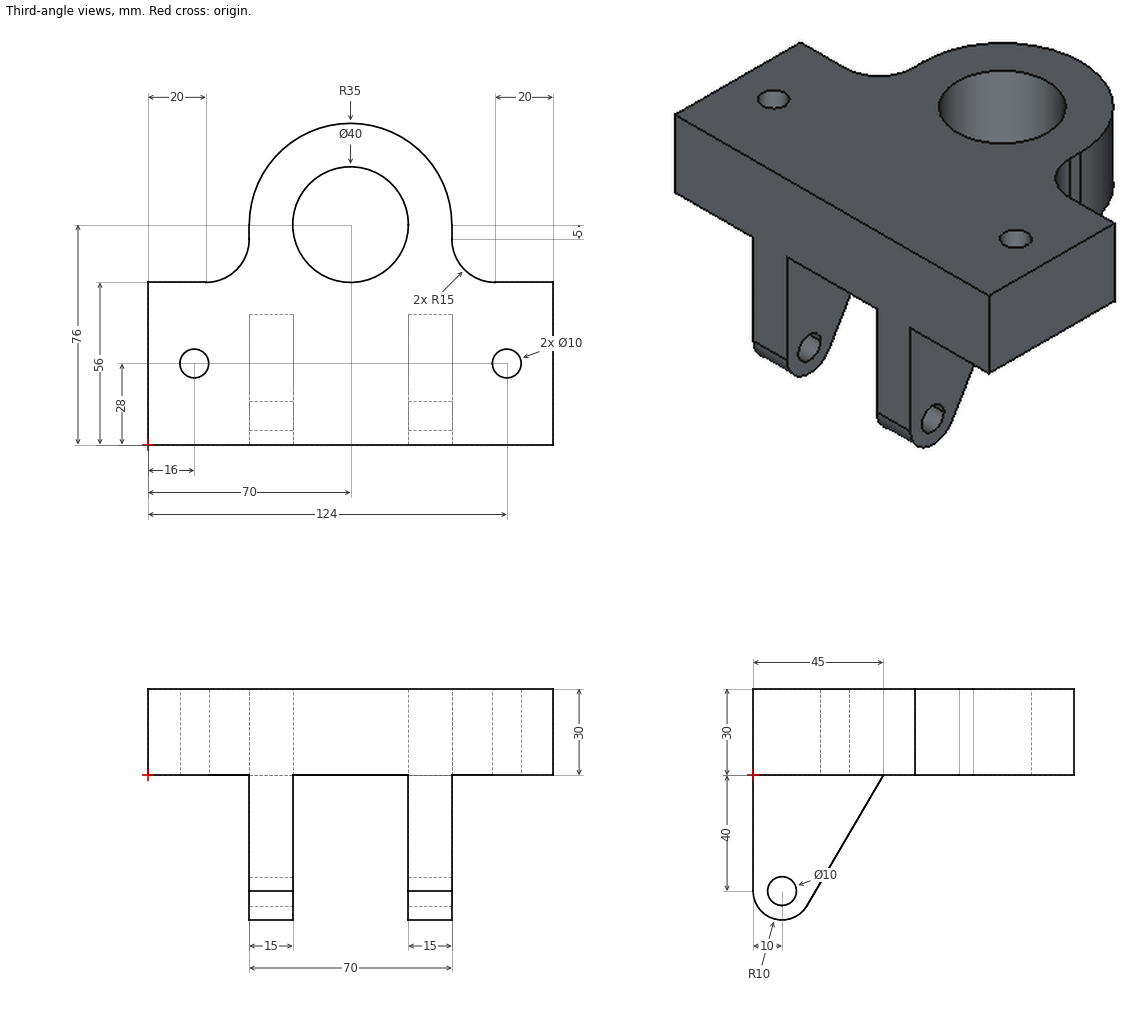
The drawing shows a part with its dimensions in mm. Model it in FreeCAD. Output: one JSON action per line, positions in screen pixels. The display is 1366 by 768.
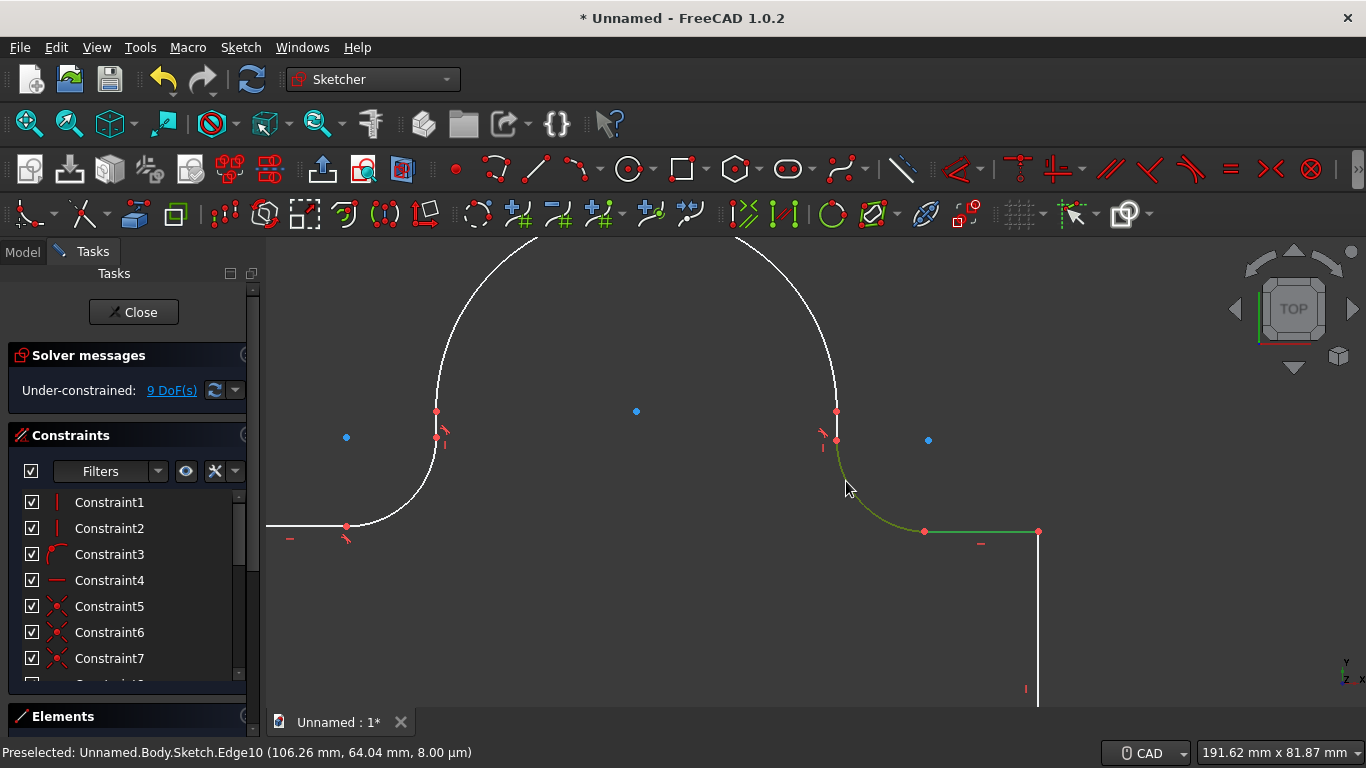
{"action": "key", "text": "t"}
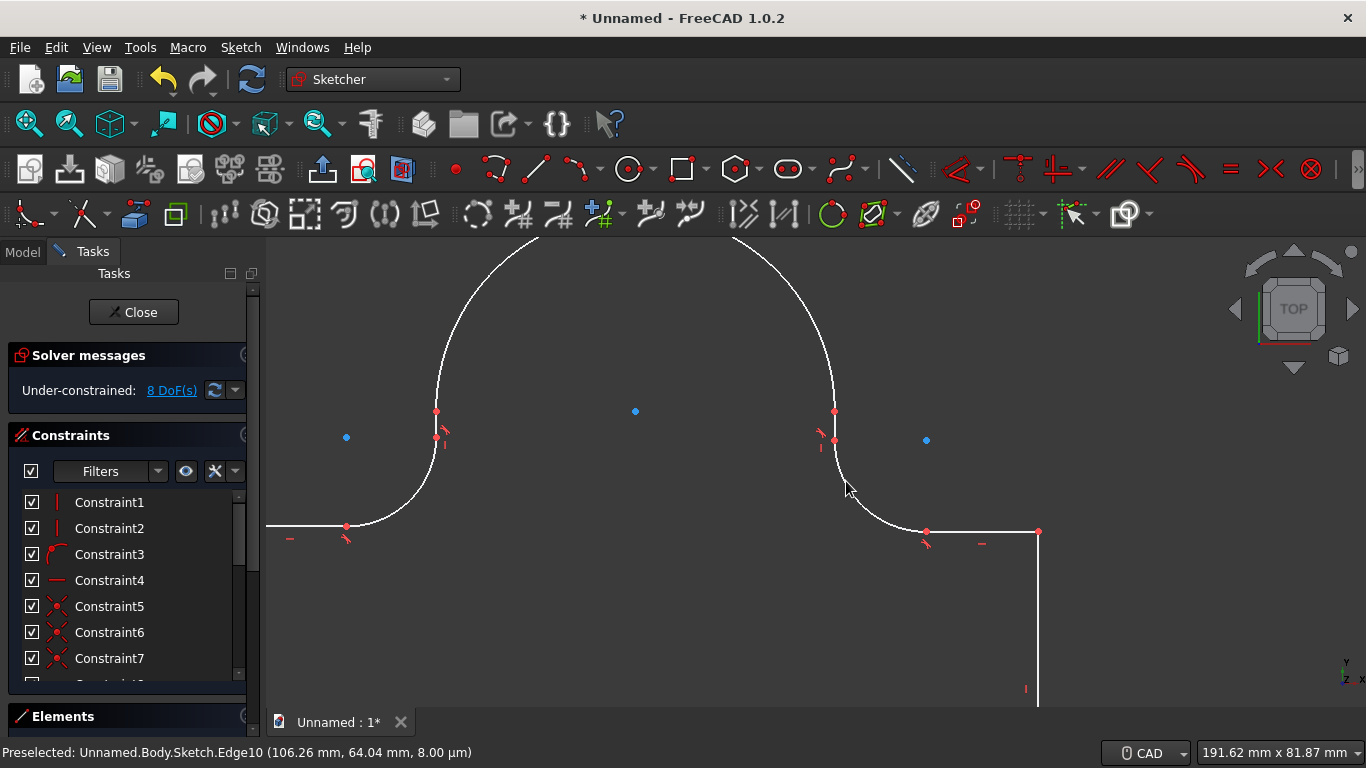
{"action": "left_click", "coordinate": [387, 517]}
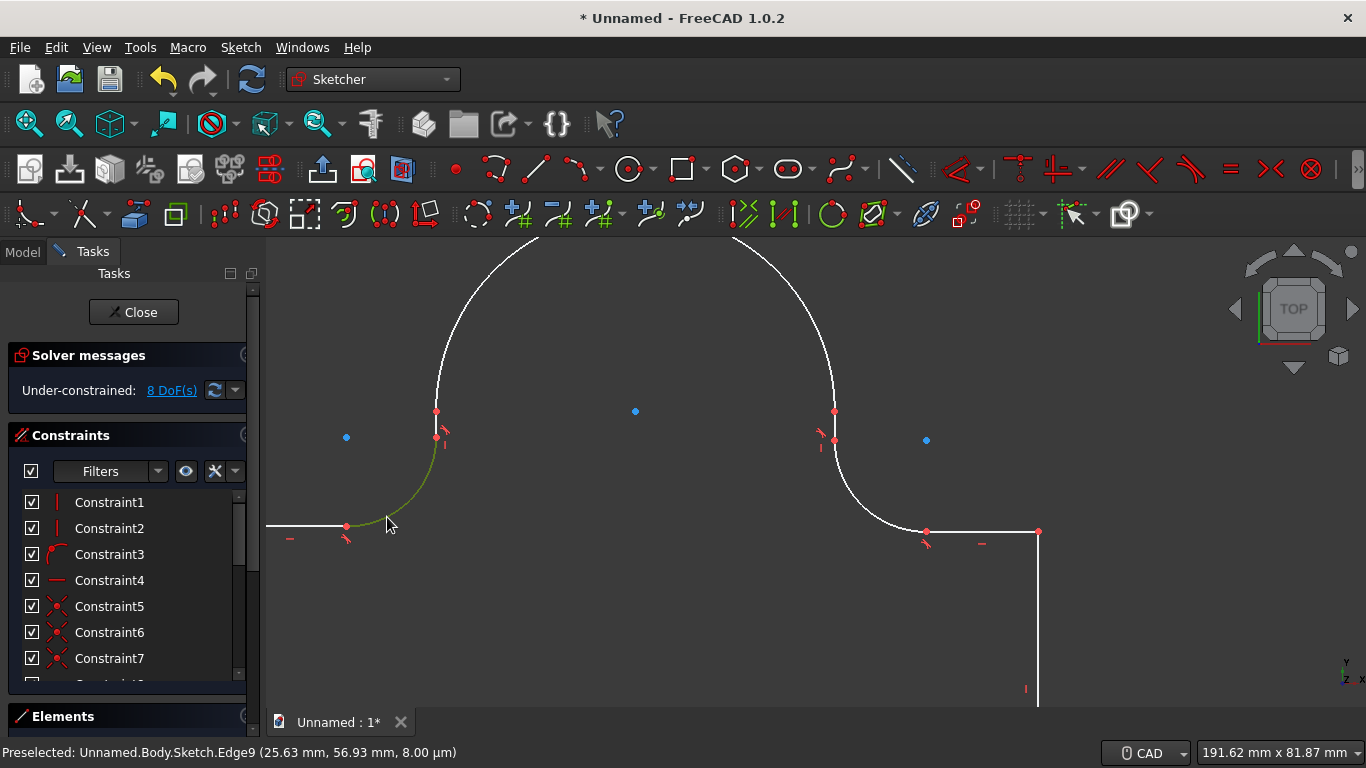
{"action": "left_click", "coordinate": [845, 482]}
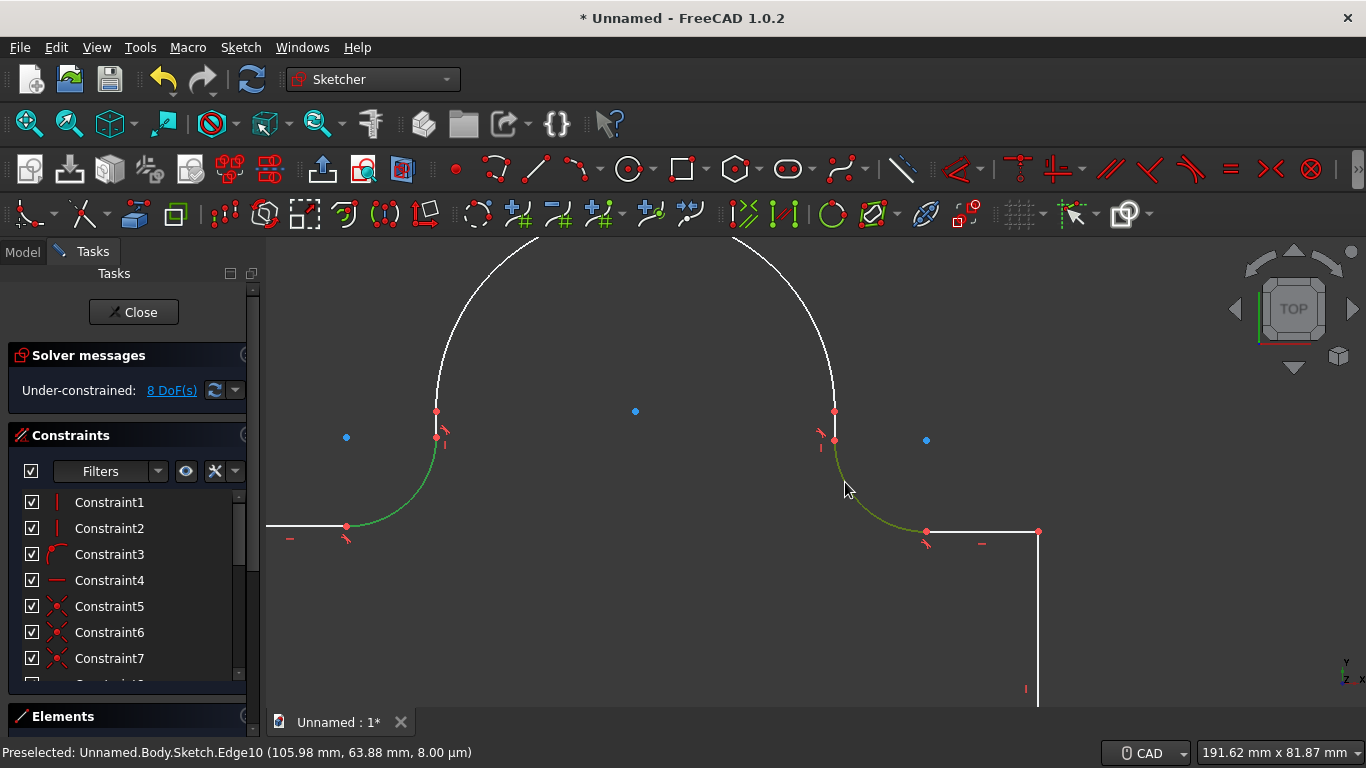
{"action": "left_click", "coordinate": [1232, 170]}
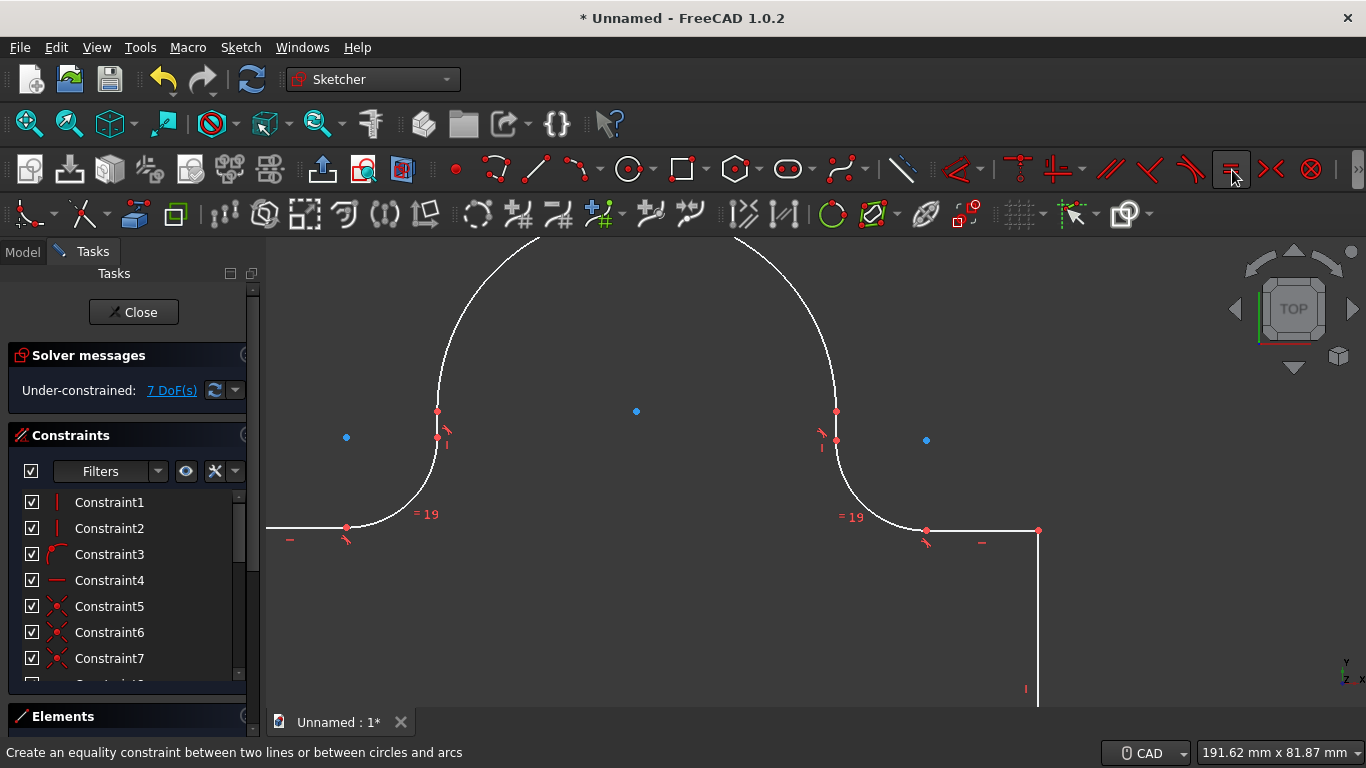
{"action": "left_click", "coordinate": [798, 294]}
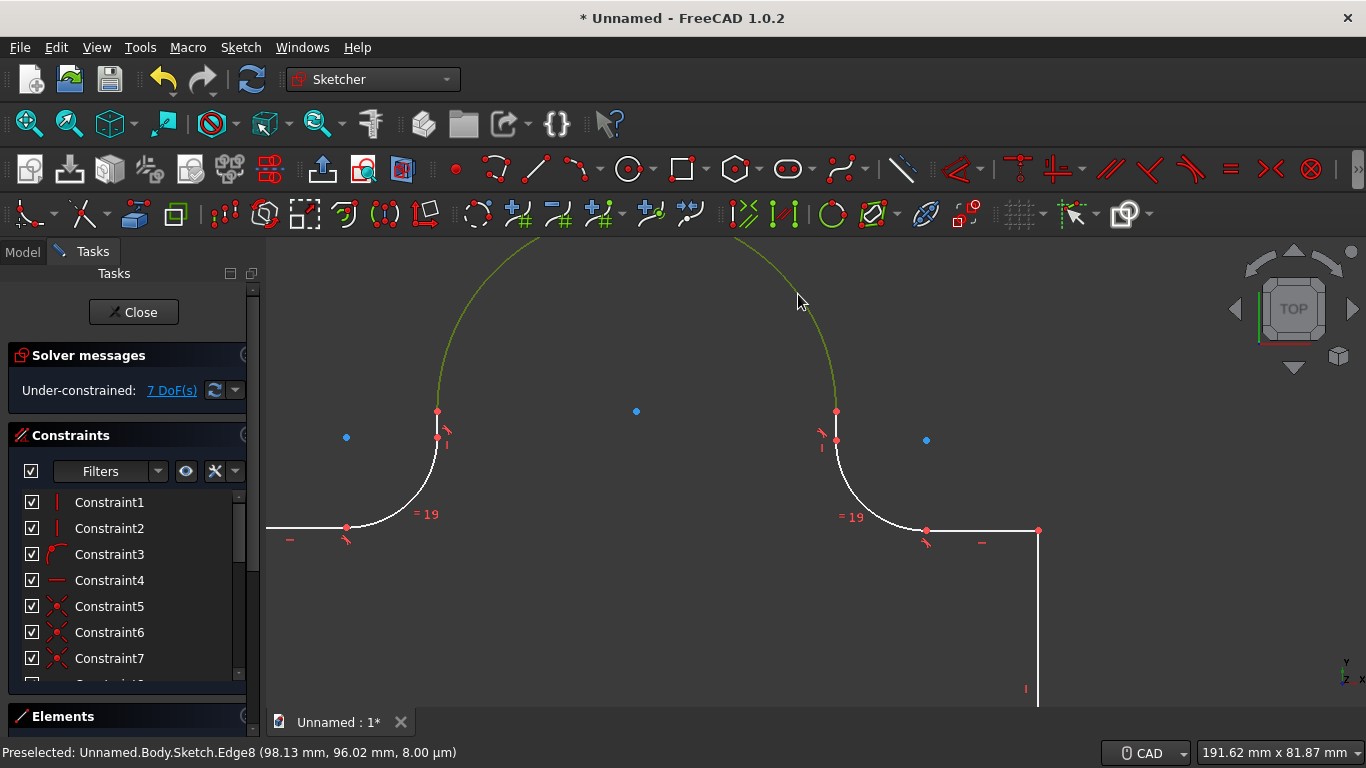
{"action": "left_click", "coordinate": [982, 170]}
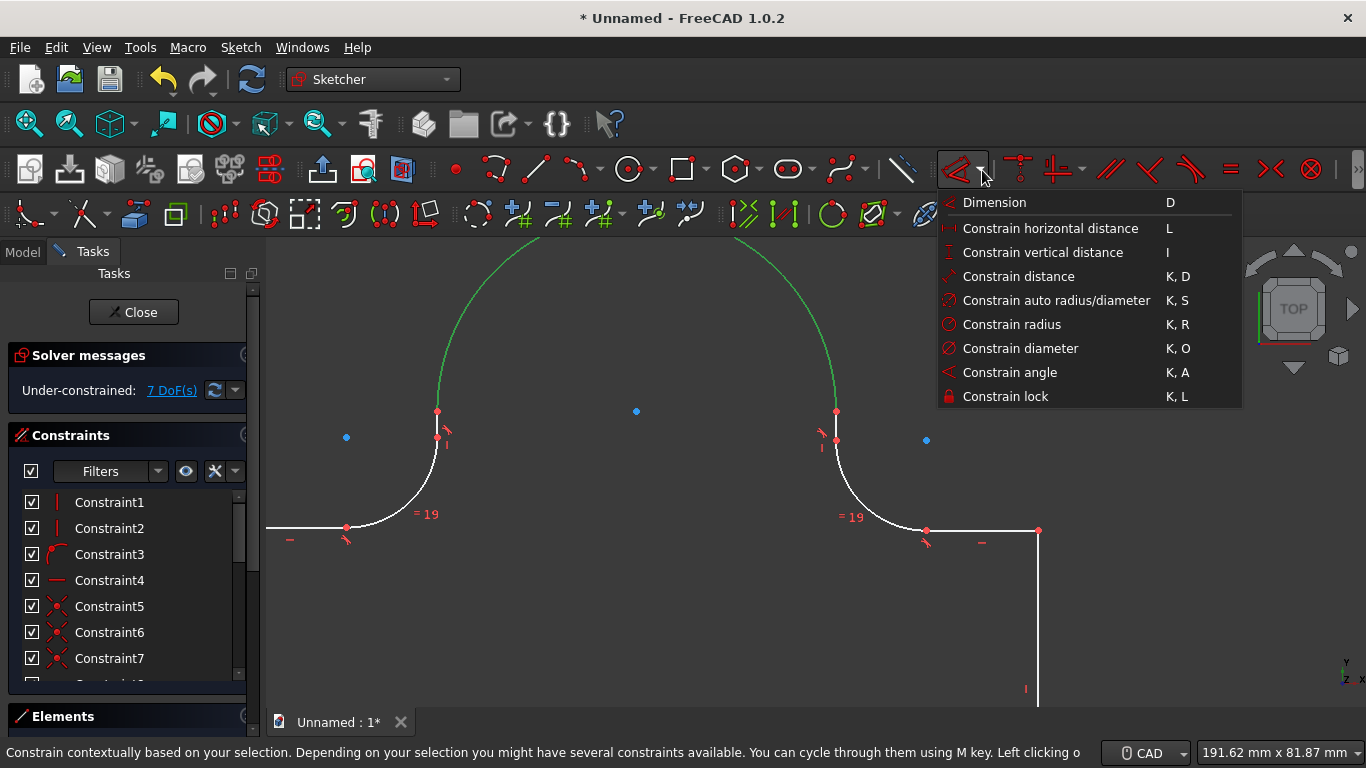
{"action": "left_click", "coordinate": [1090, 324]}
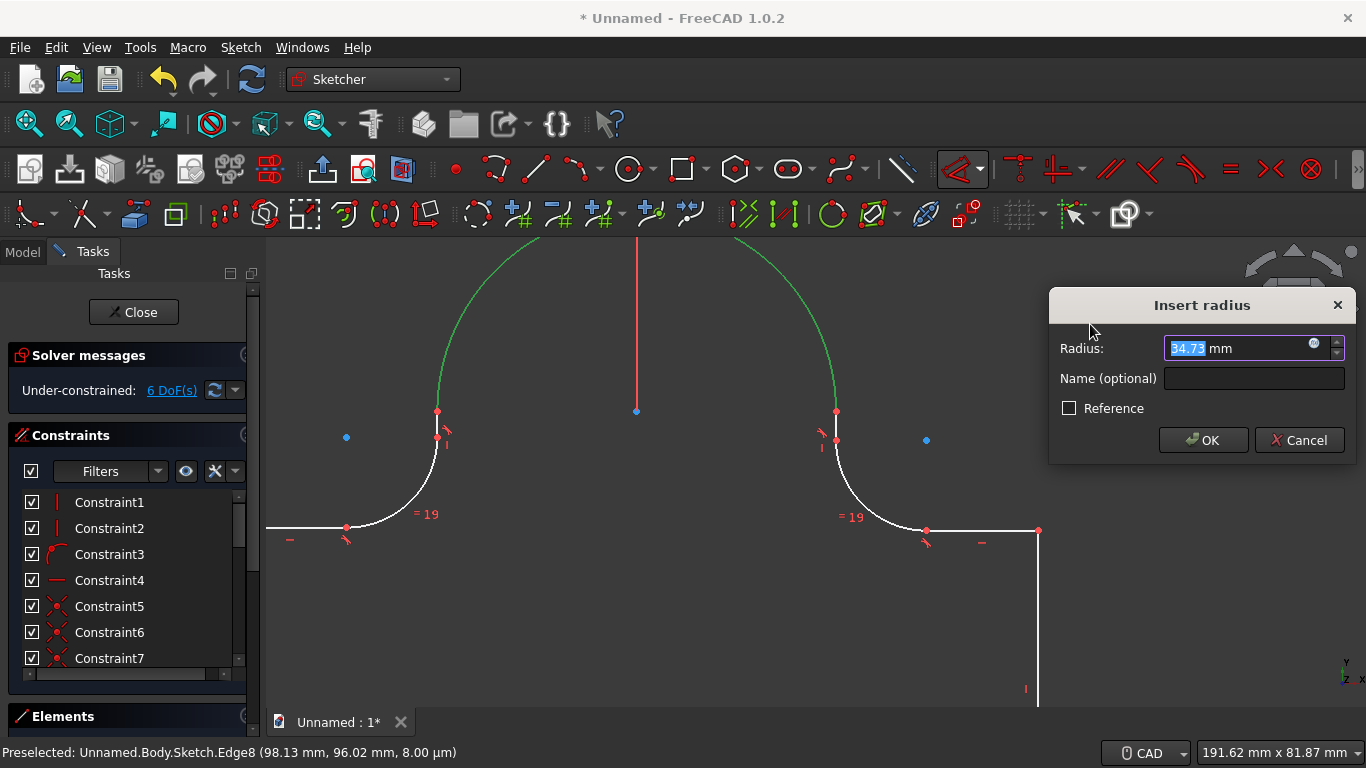
{"action": "type", "text": "35"}
{"action": "key", "text": "Return"}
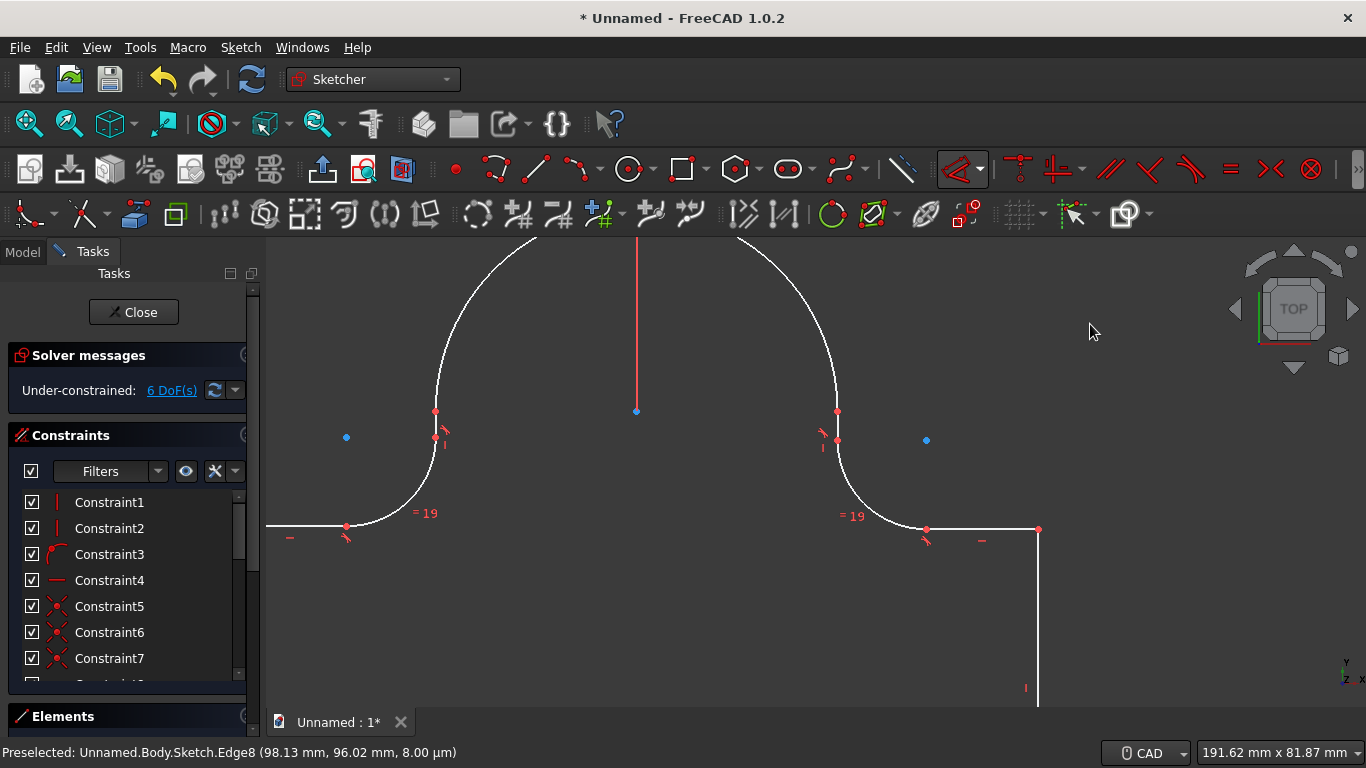
{"action": "left_click", "coordinate": [387, 516]}